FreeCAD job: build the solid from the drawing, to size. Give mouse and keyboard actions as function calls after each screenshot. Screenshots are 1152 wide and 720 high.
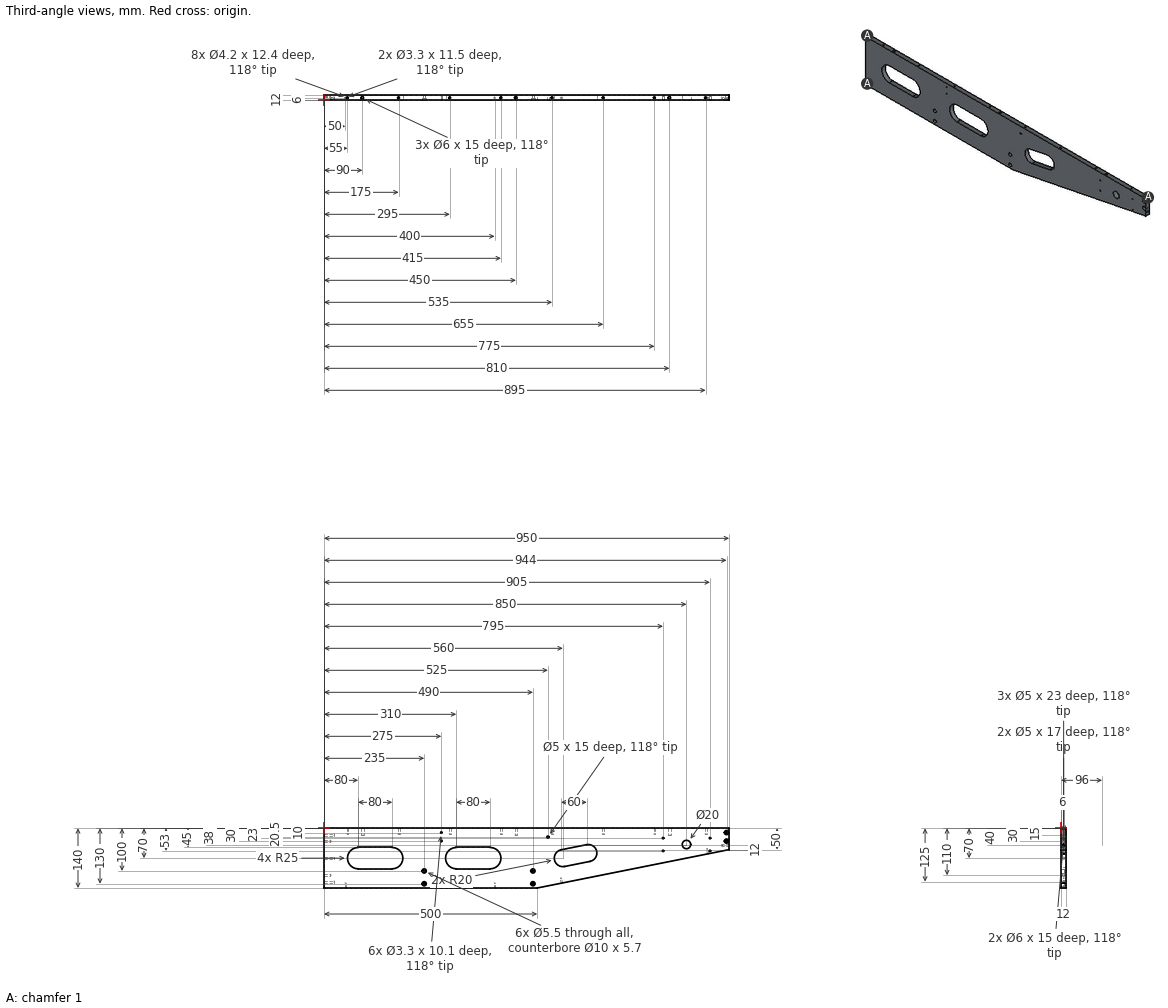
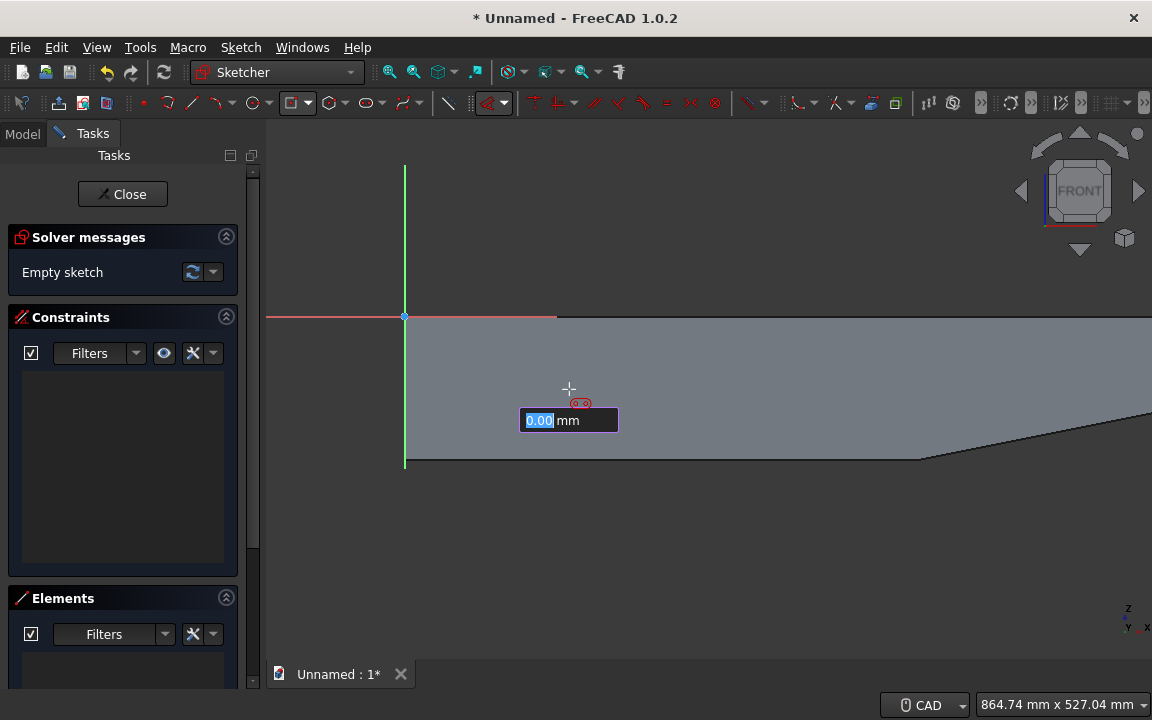
click(528, 363)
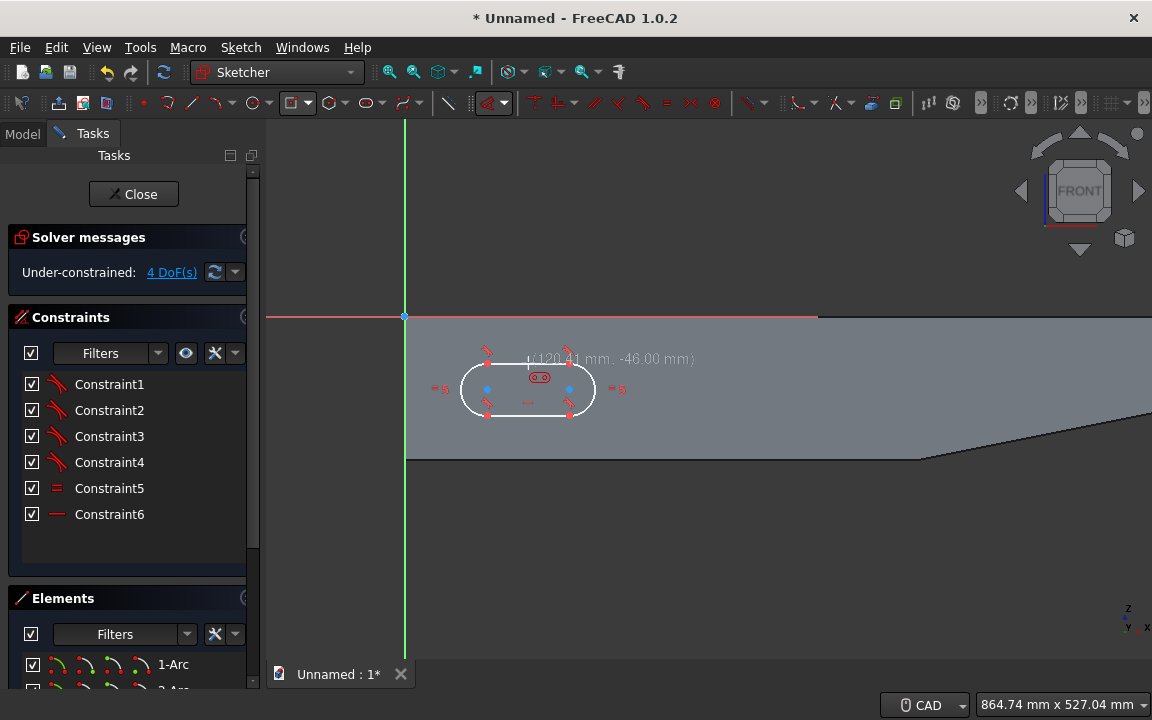
click(722, 389)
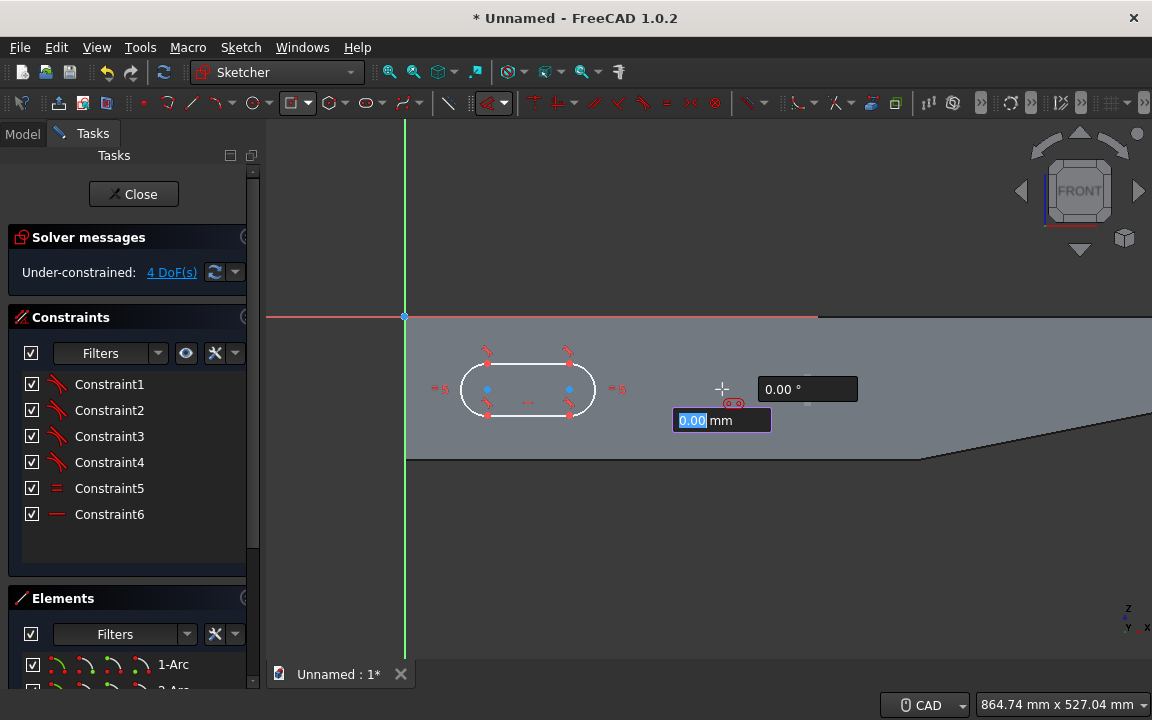
click(804, 389)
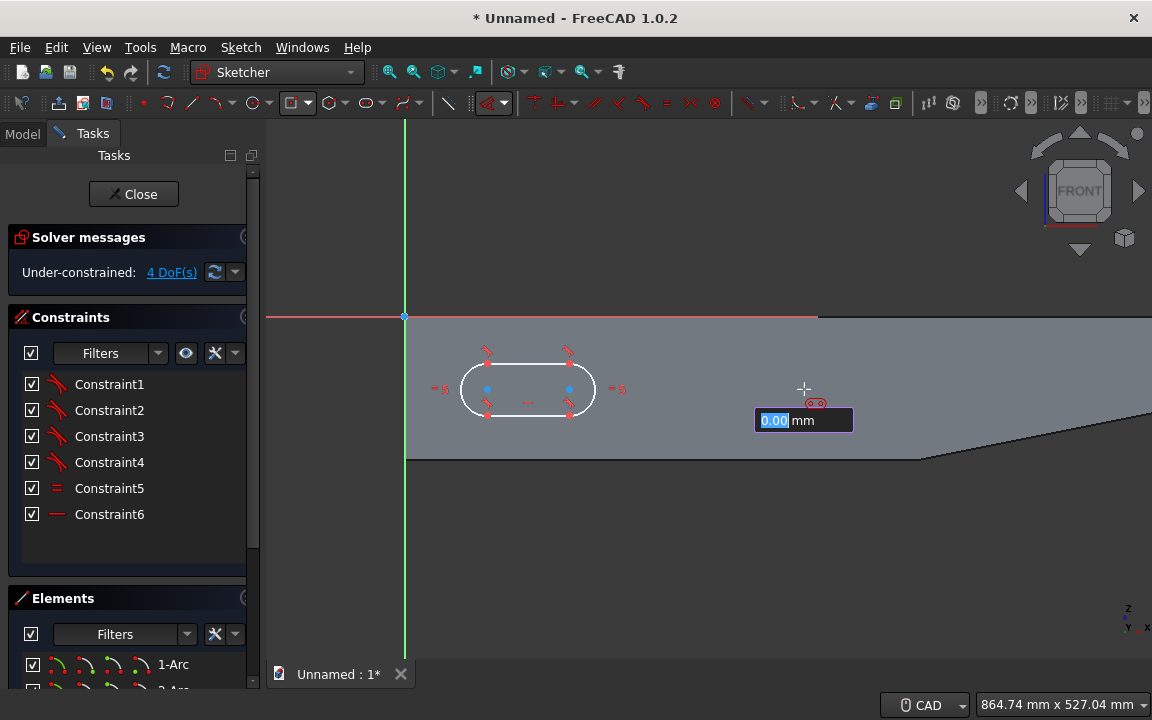
click(763, 363)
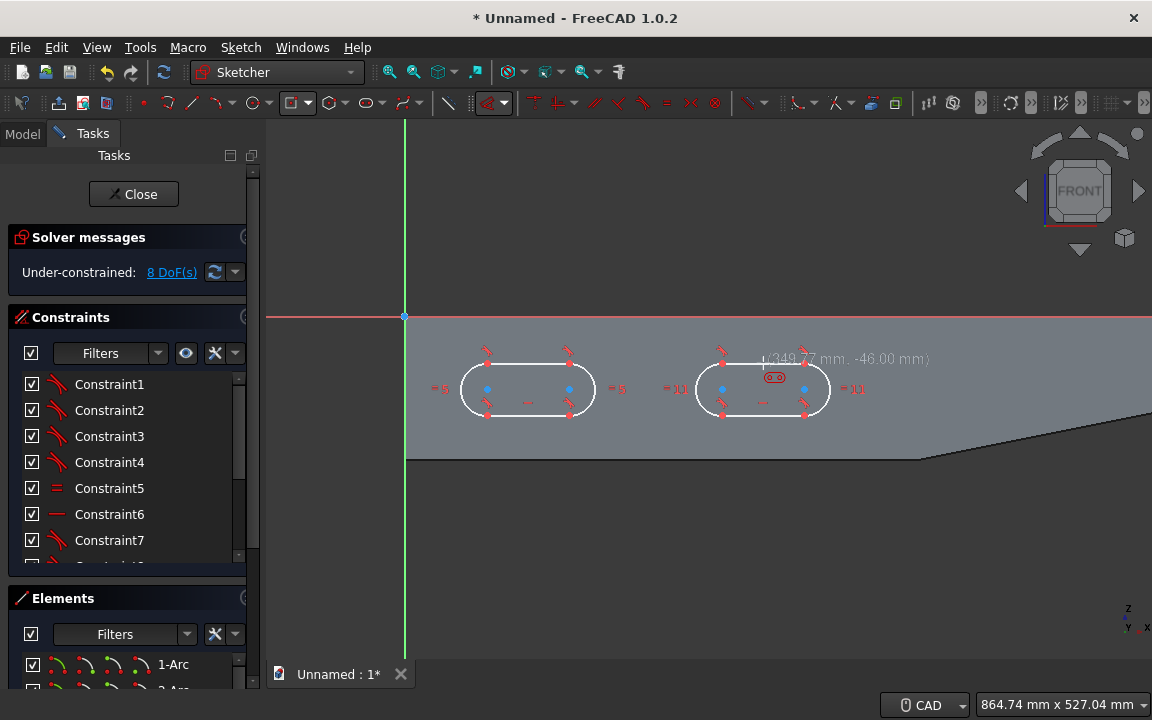
click(978, 389)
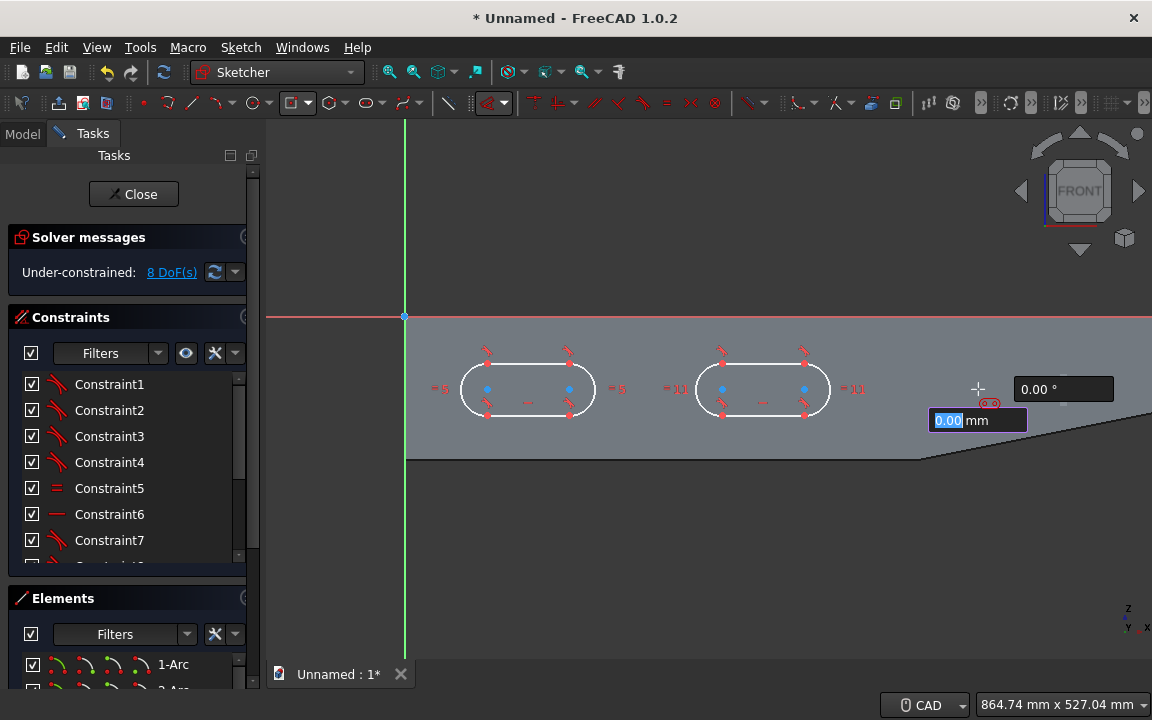
scroll(392, 418, down, 3)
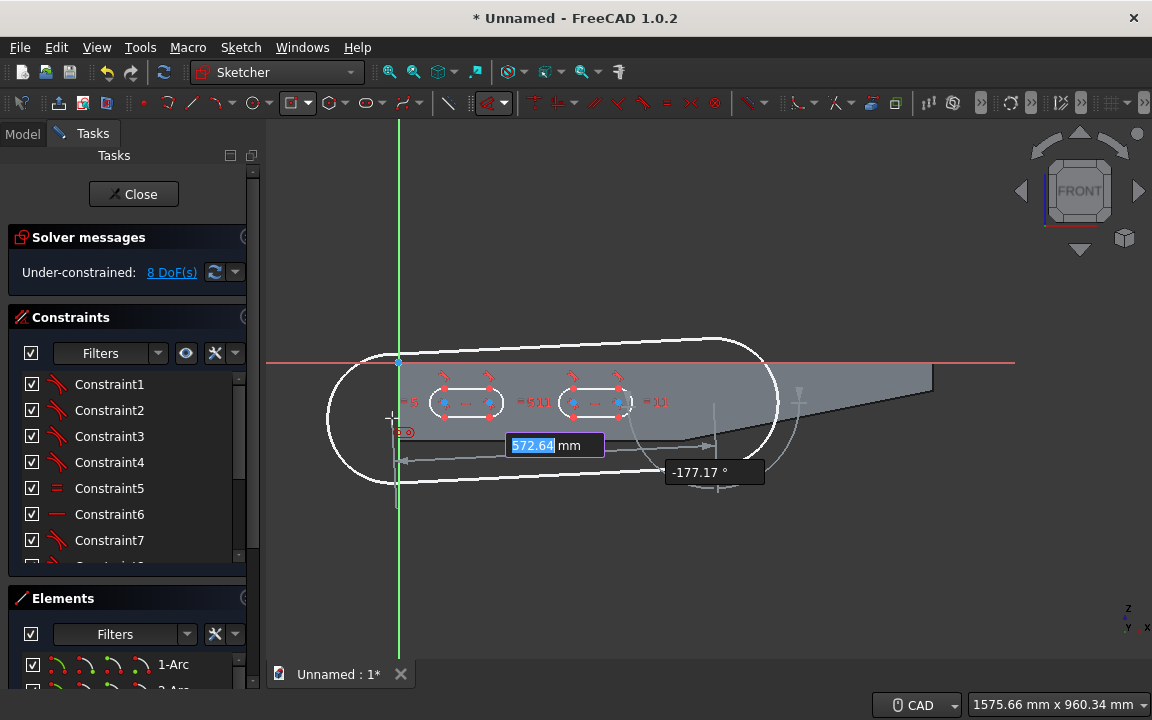
click(748, 395)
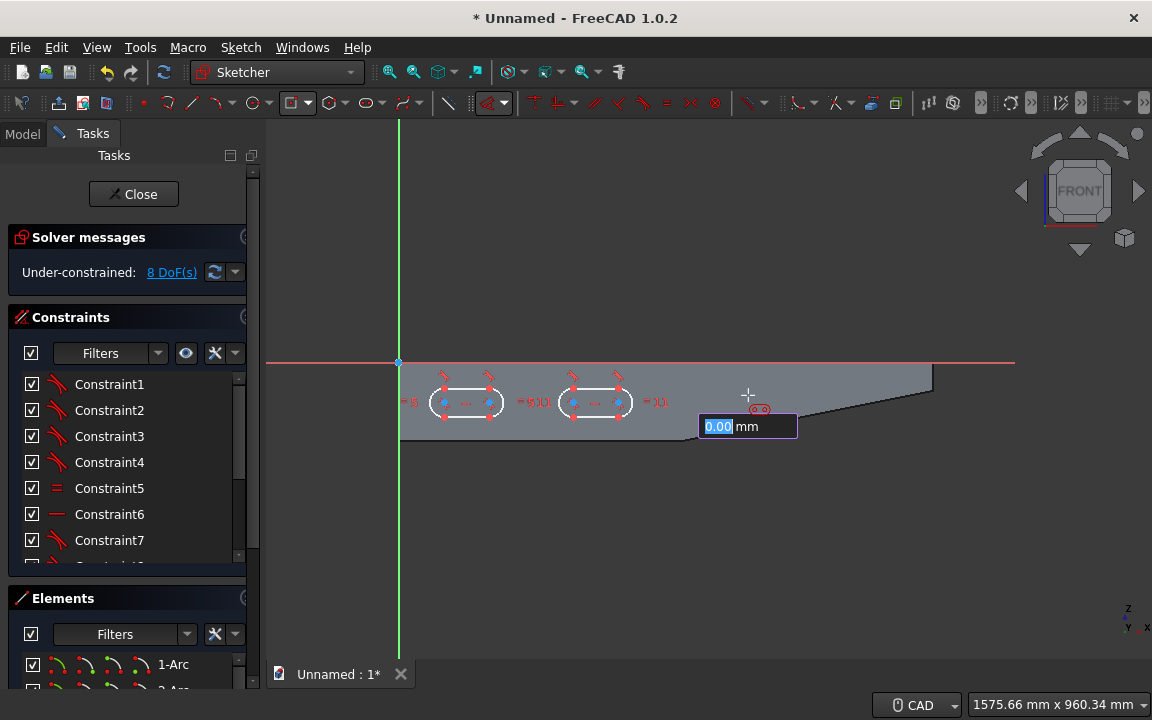
scroll(729, 388, up, 2)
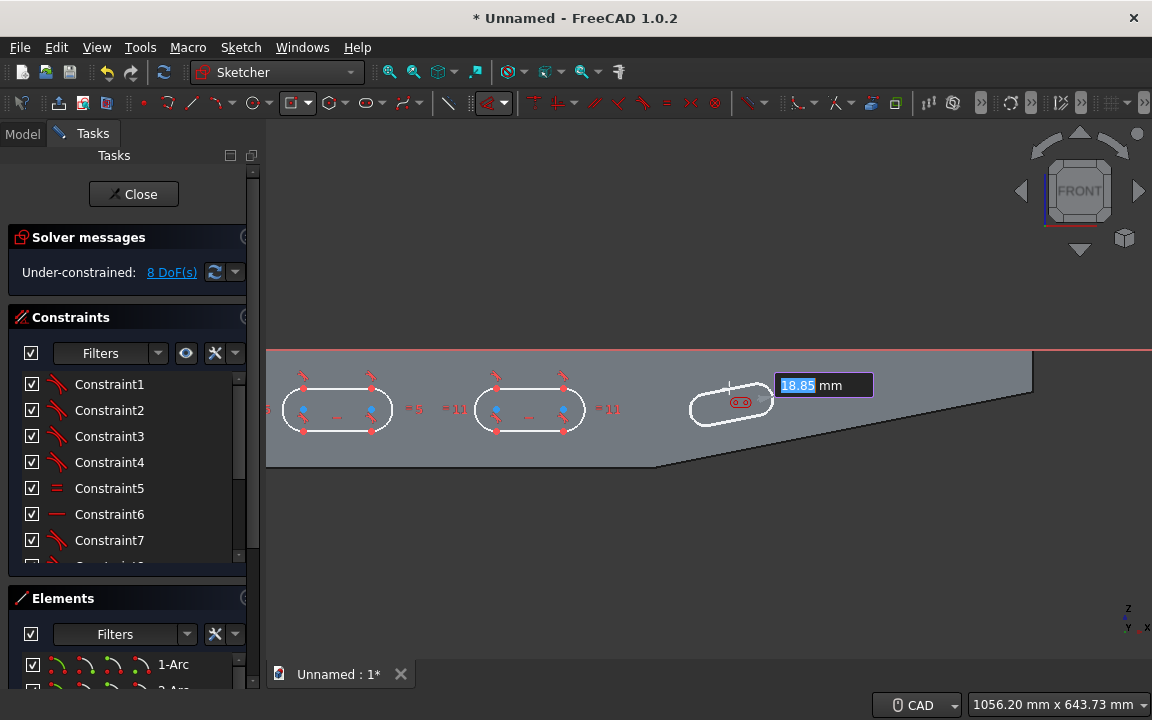
click(728, 387)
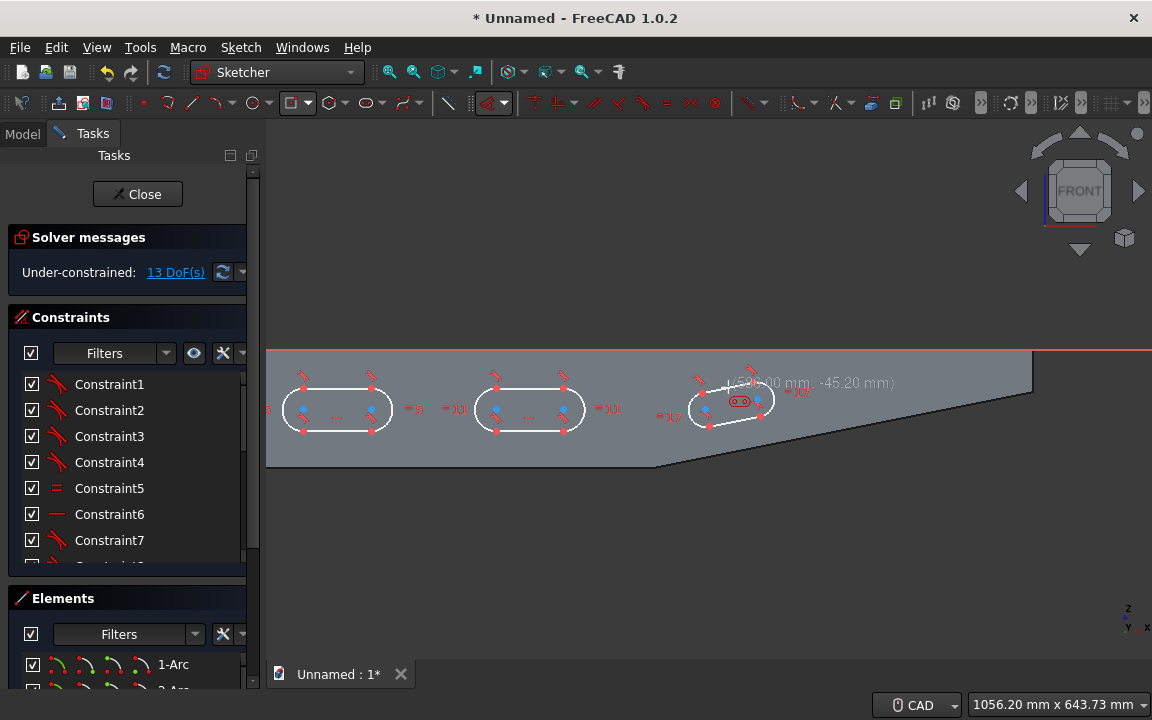
click(254, 104)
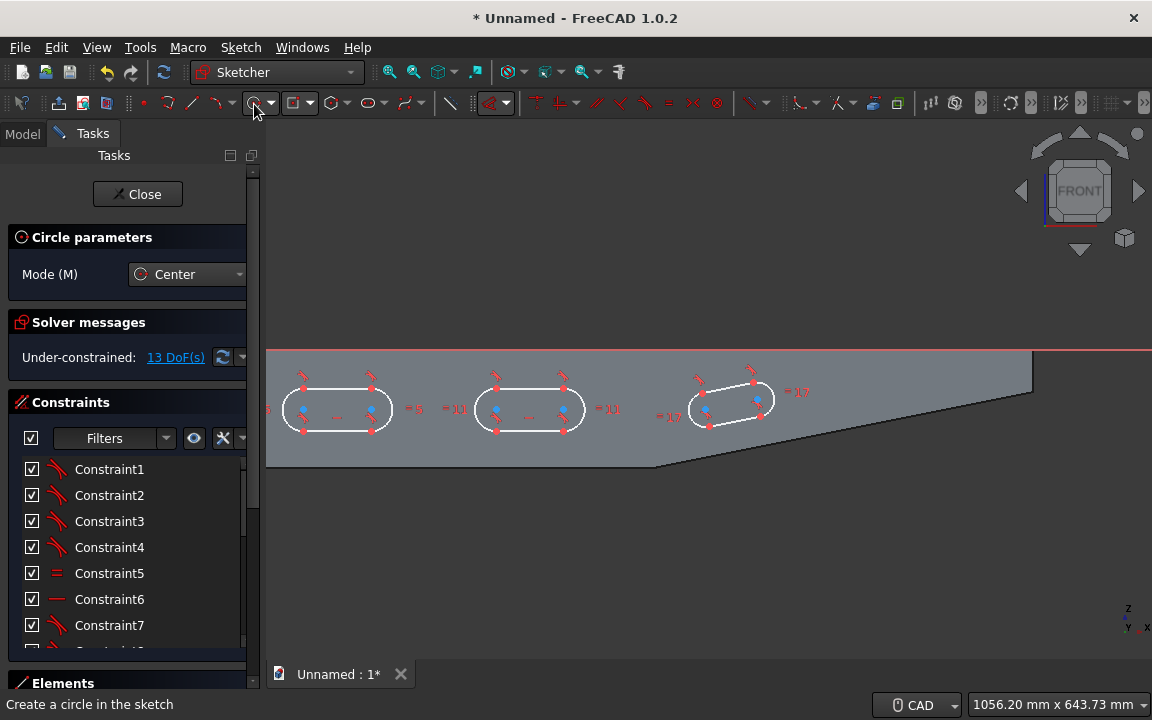
scroll(949, 382, up, 5)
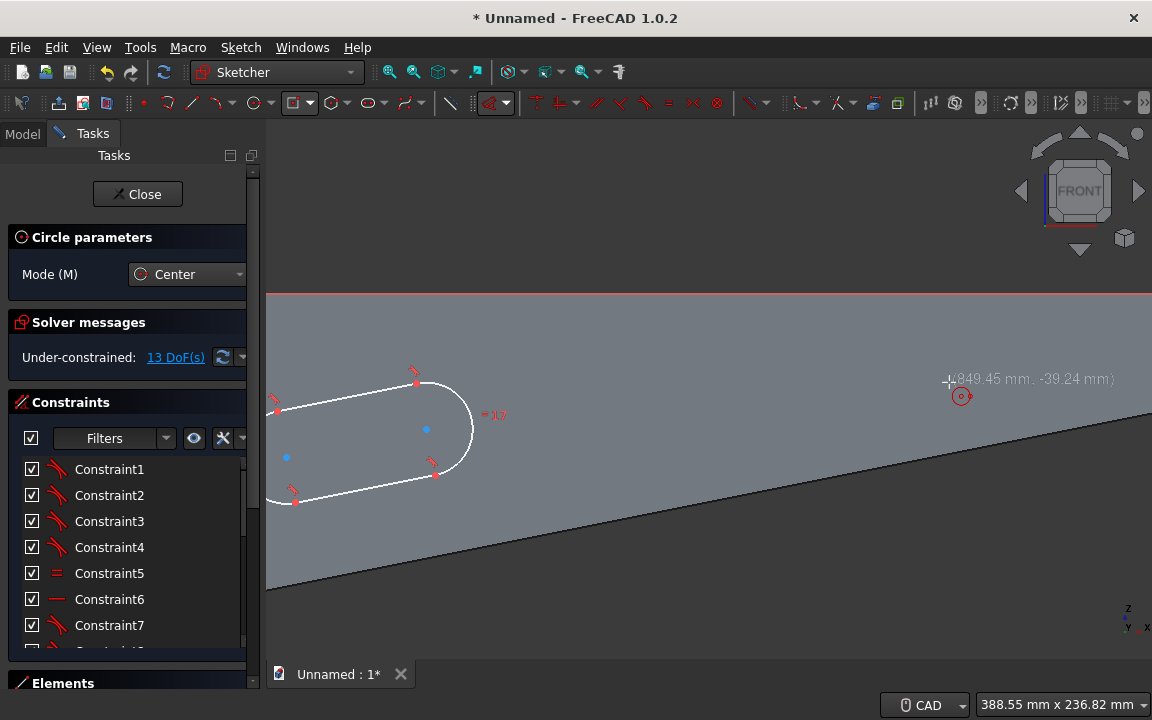
scroll(853, 385, down, 7)